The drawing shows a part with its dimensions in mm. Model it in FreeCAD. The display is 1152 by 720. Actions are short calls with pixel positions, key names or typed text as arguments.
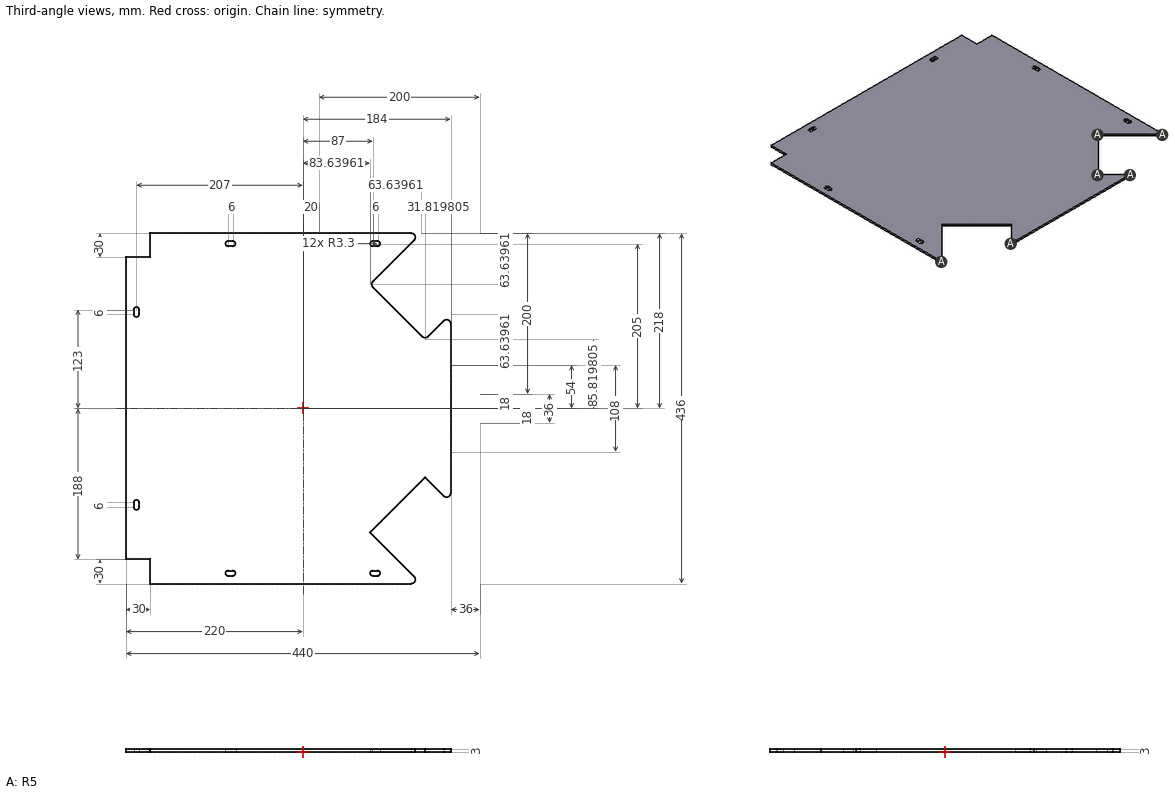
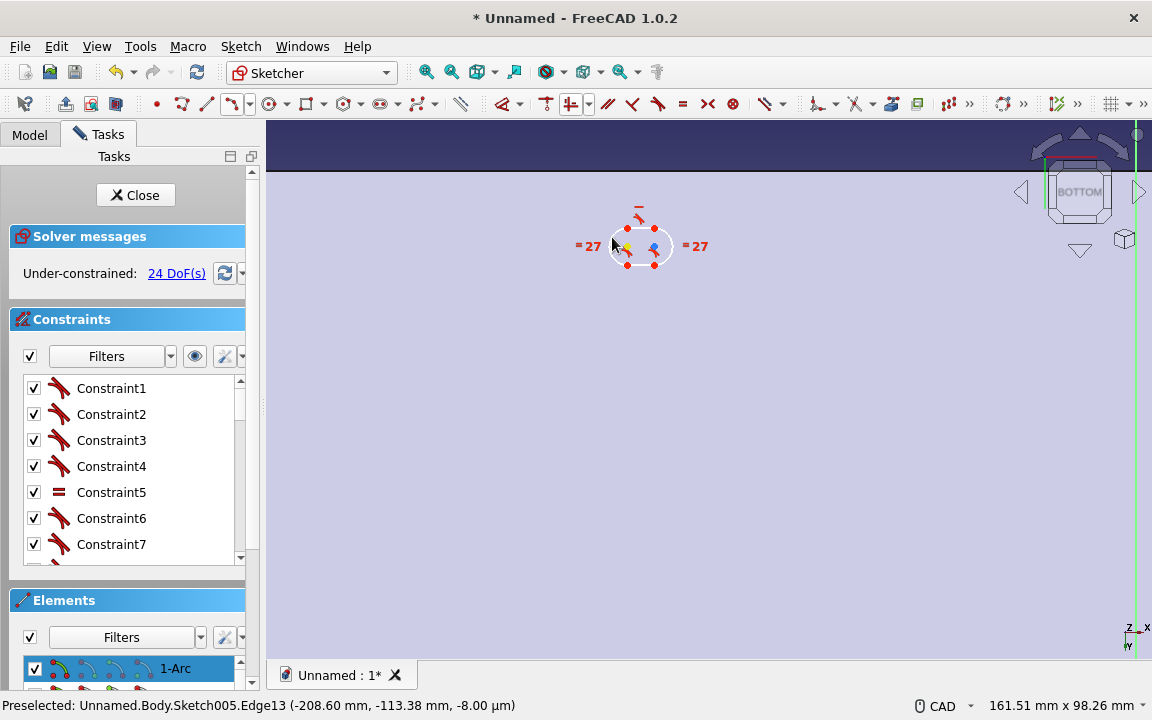
click(613, 236)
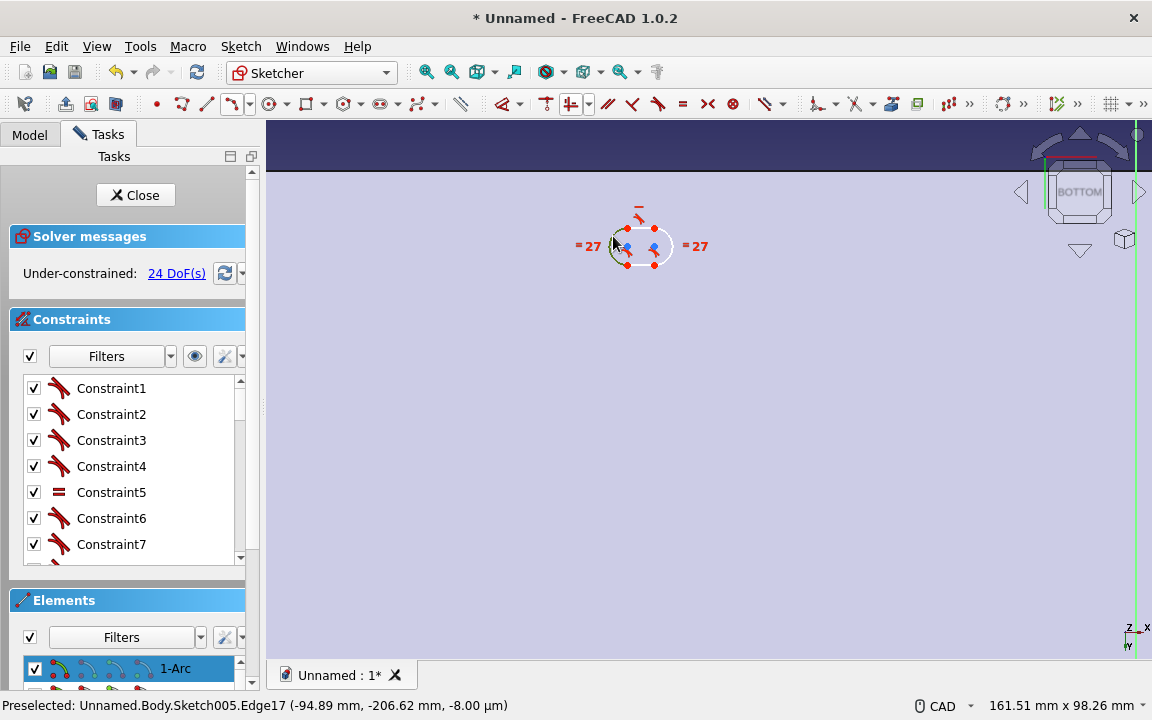
scroll(612, 237, down, 10)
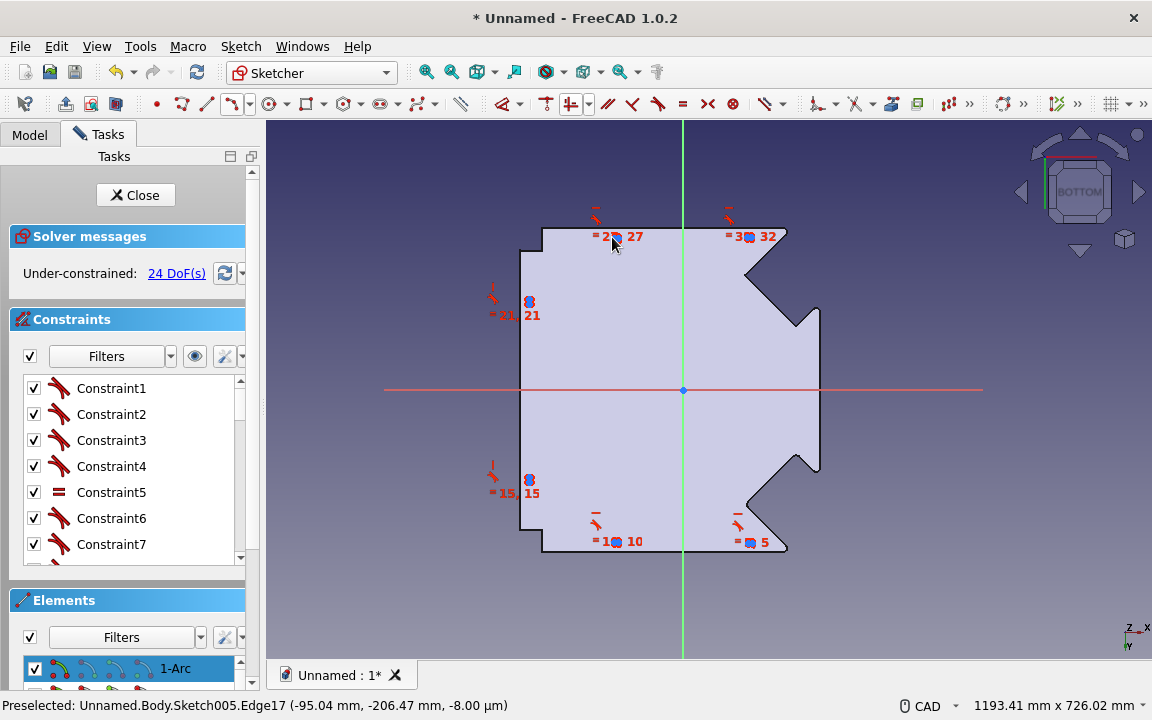
scroll(746, 236, up, 10)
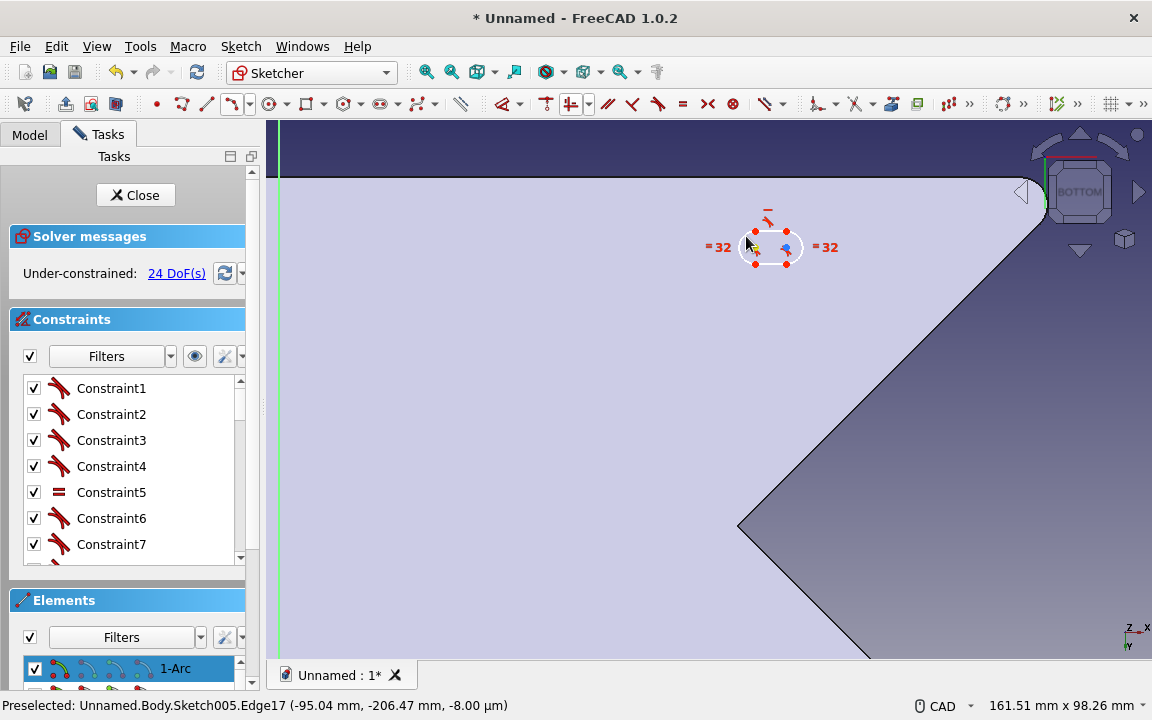
click(742, 238)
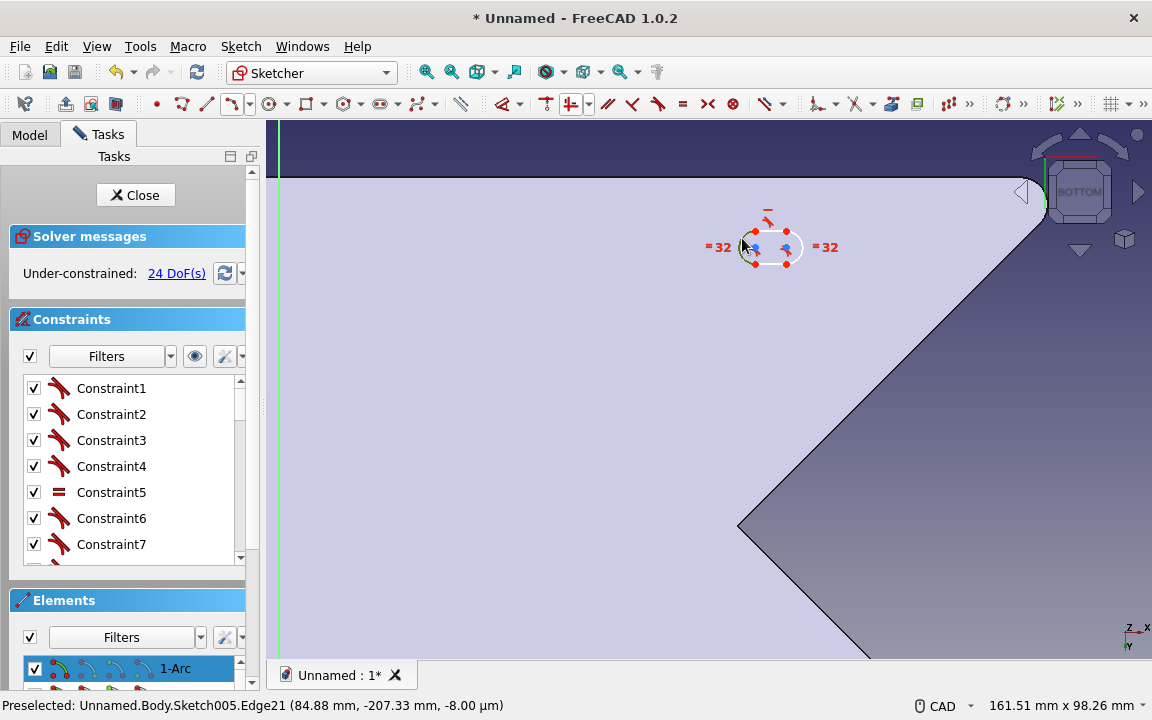
key(e)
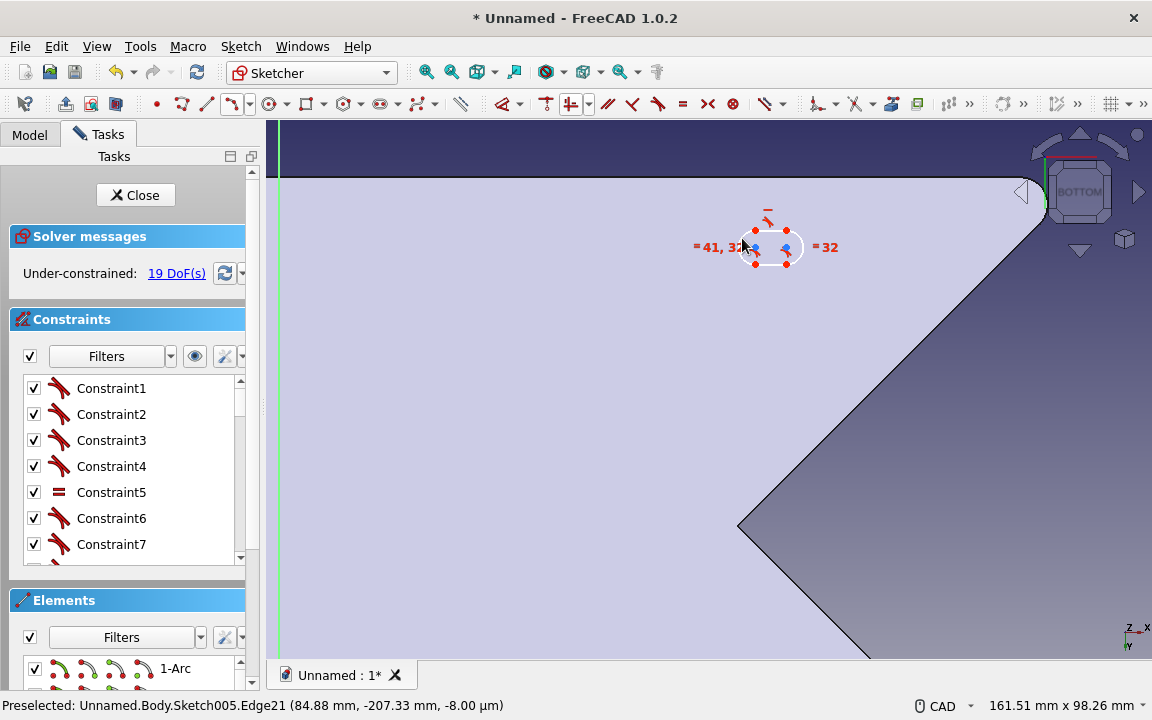
scroll(746, 236, down, 10)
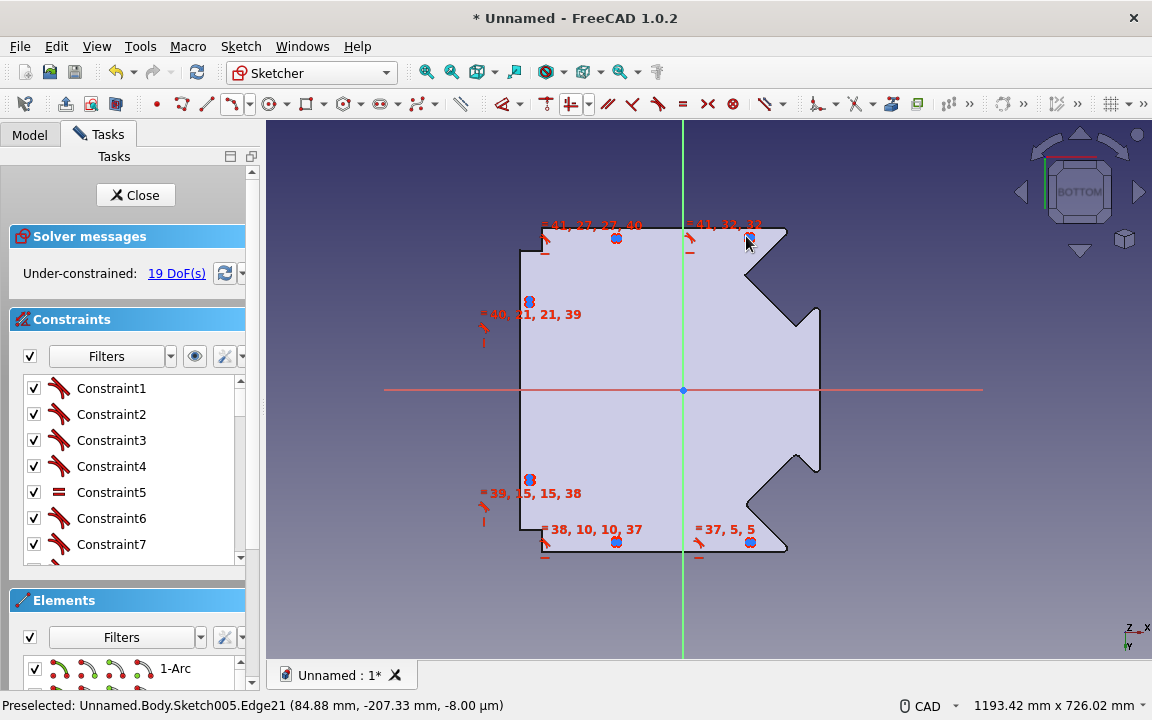
scroll(752, 542, up, 9)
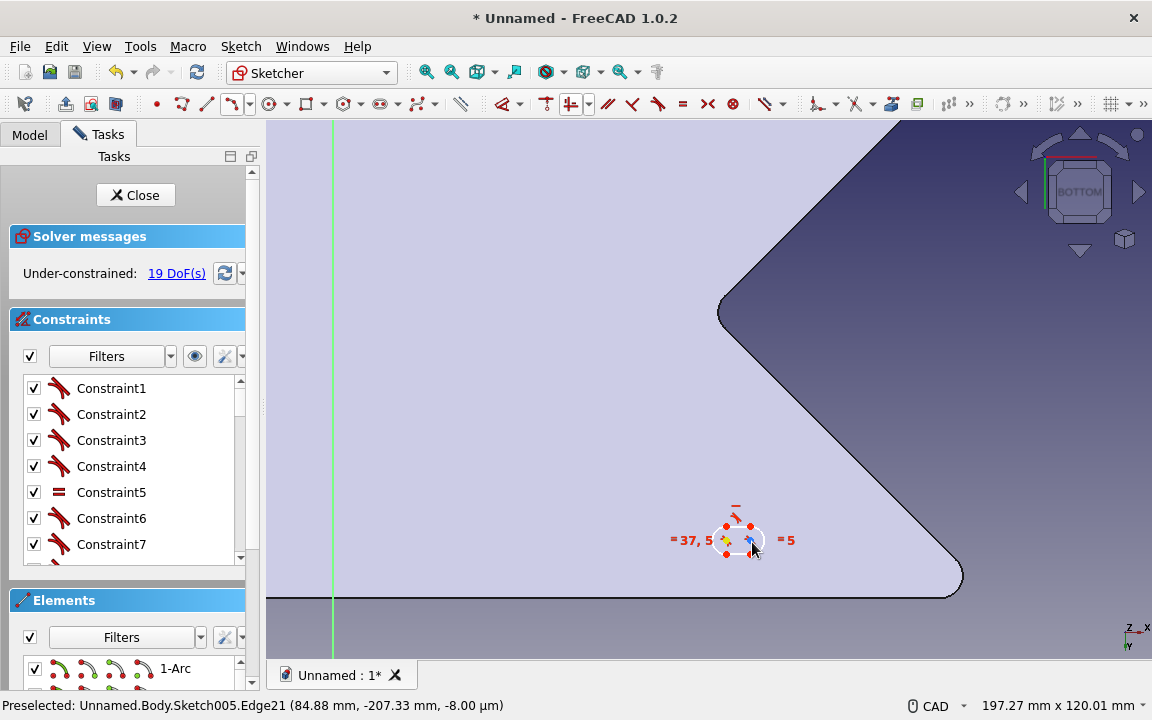
click(750, 541)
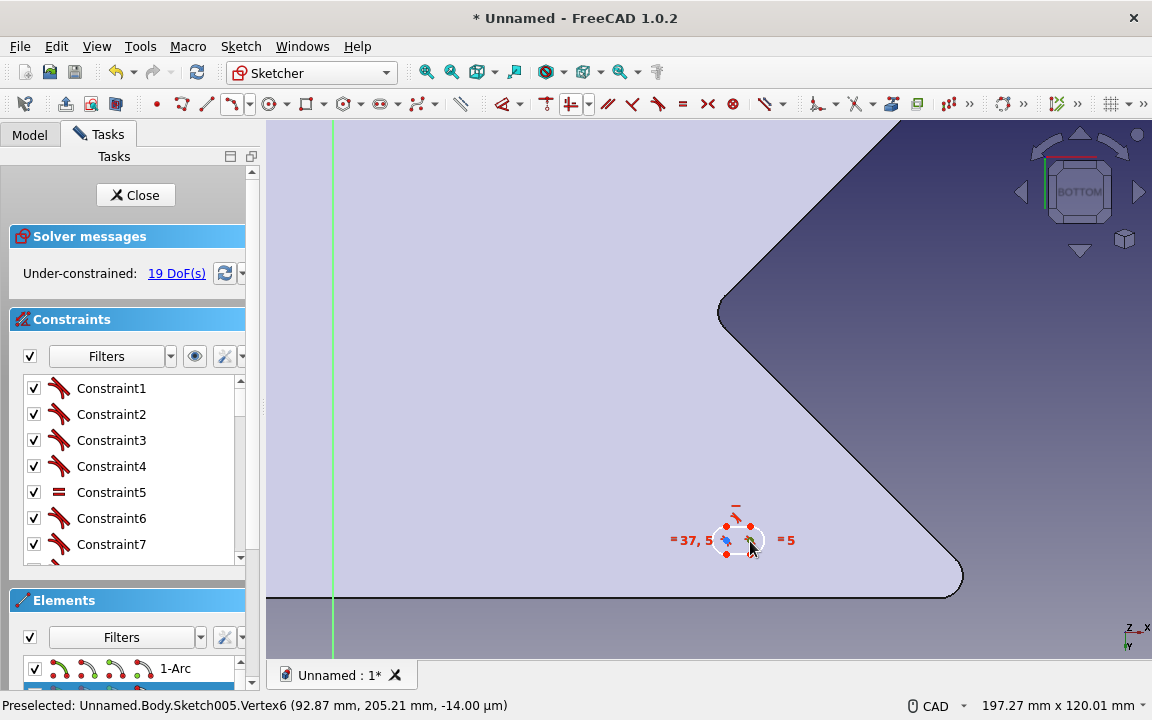
scroll(752, 542, down, 9)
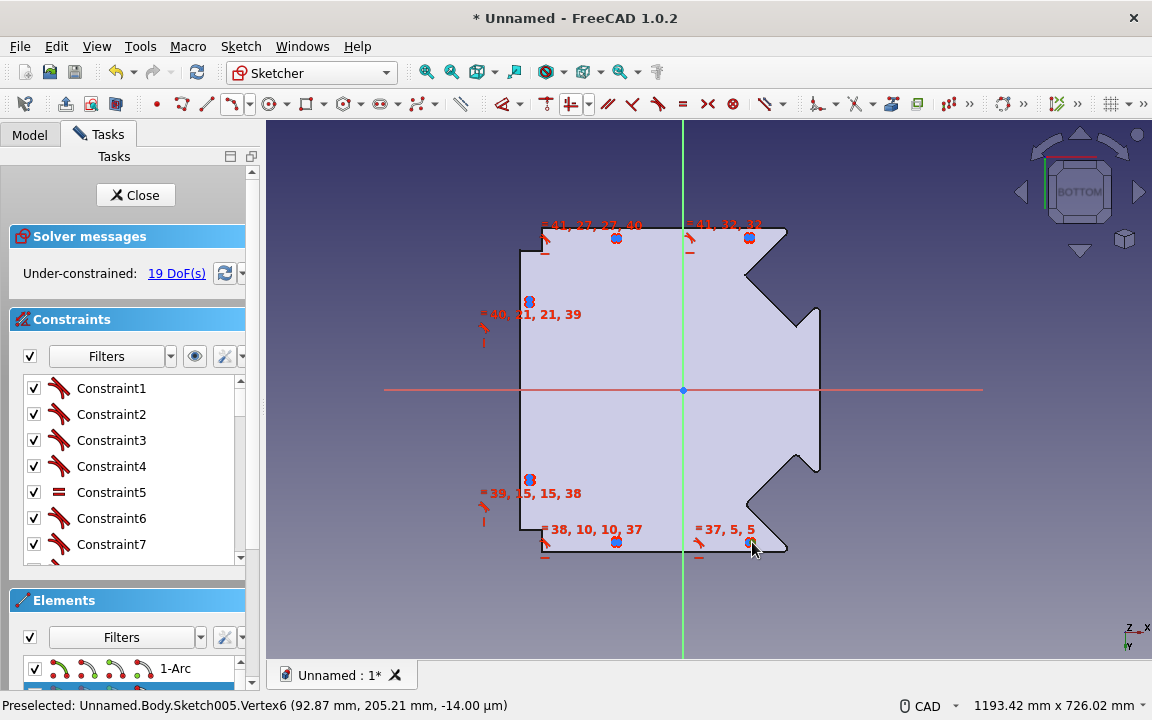
scroll(614, 542, up, 9)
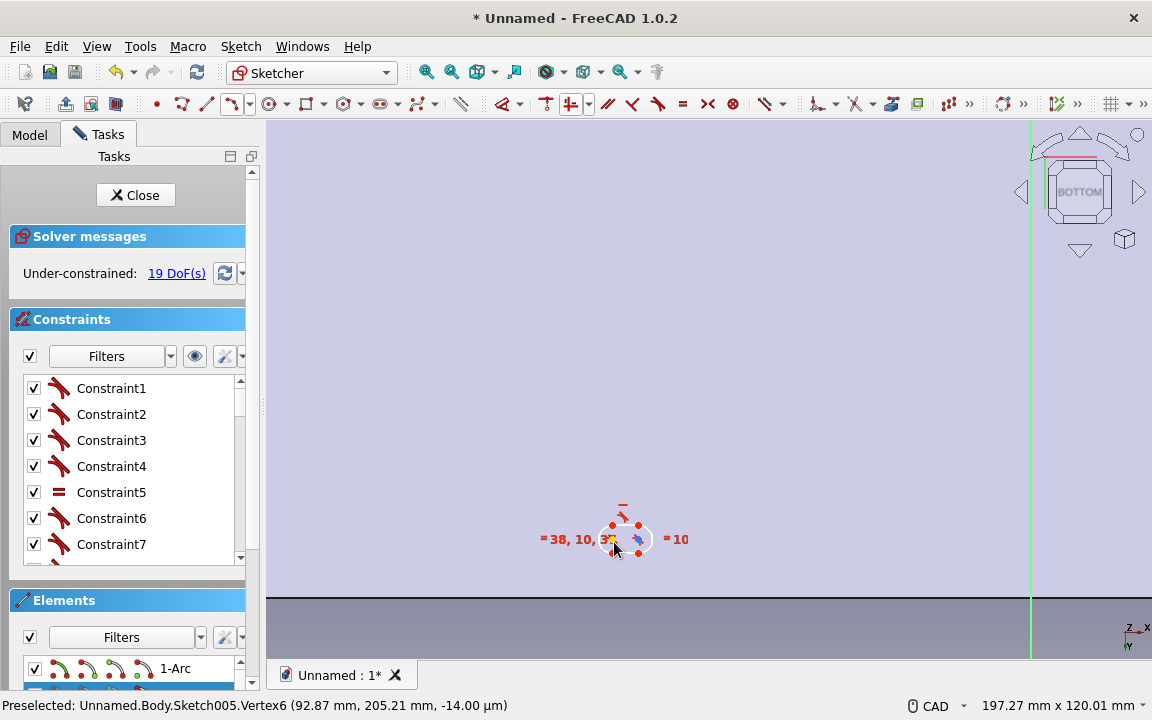
click(613, 539)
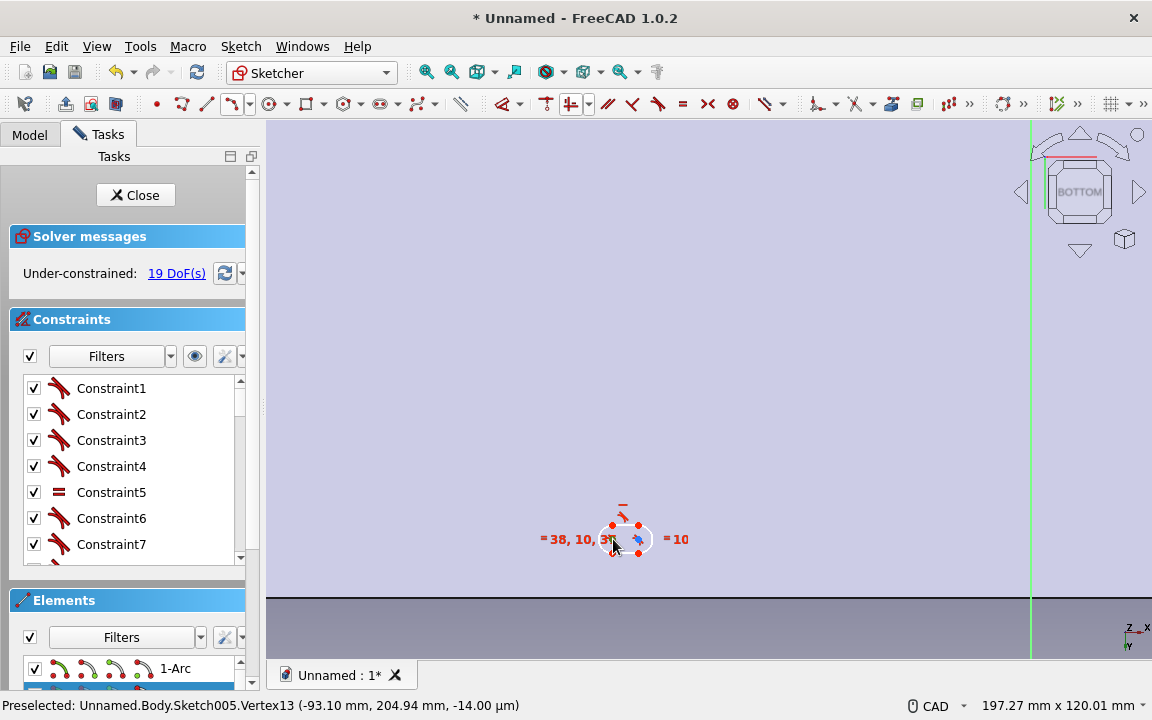
scroll(614, 542, down, 9)